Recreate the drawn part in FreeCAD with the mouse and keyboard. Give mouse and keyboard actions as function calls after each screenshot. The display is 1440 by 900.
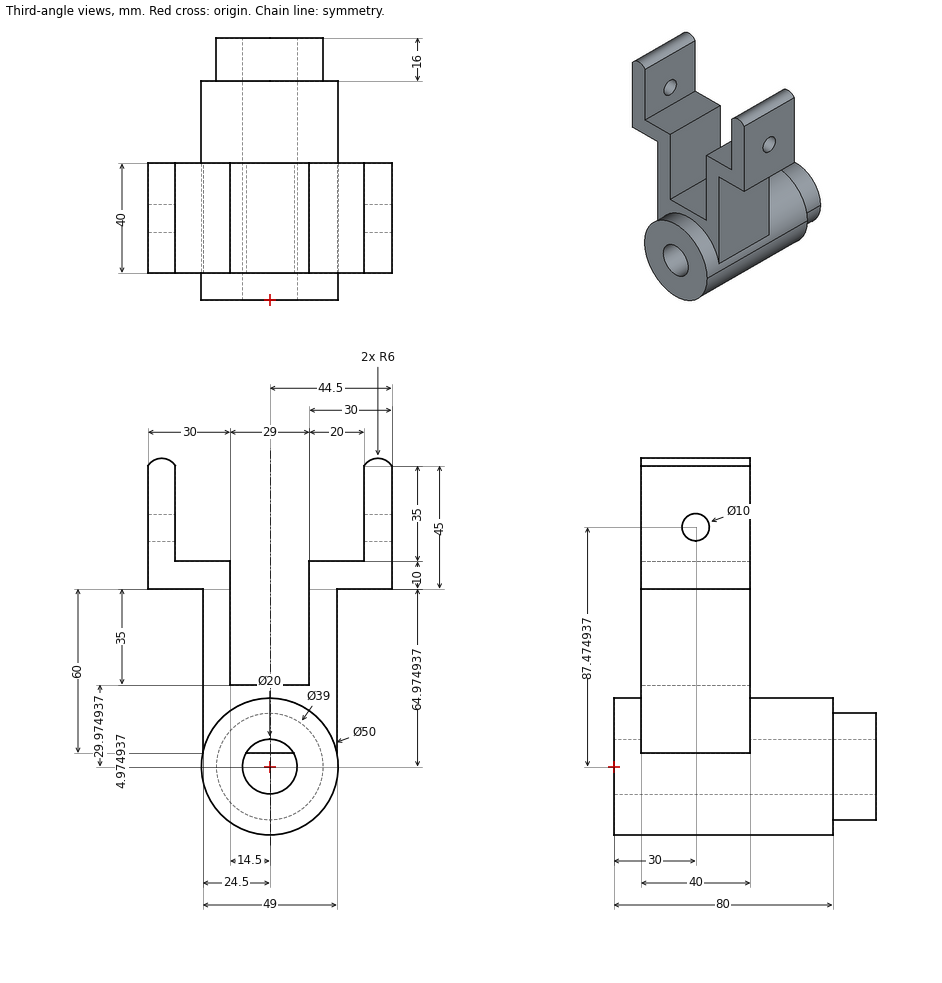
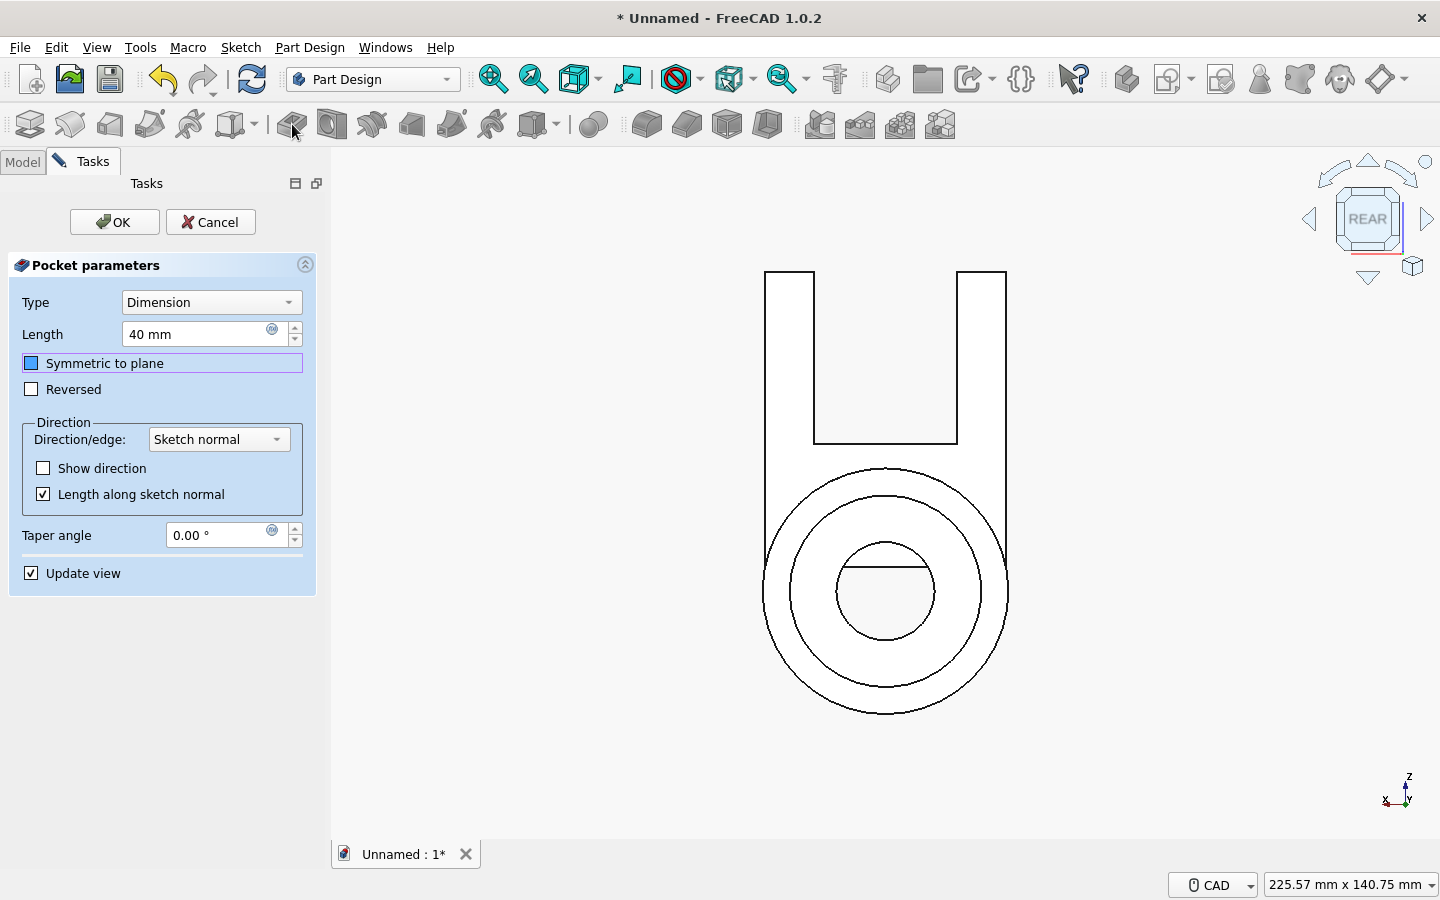
click(115, 222)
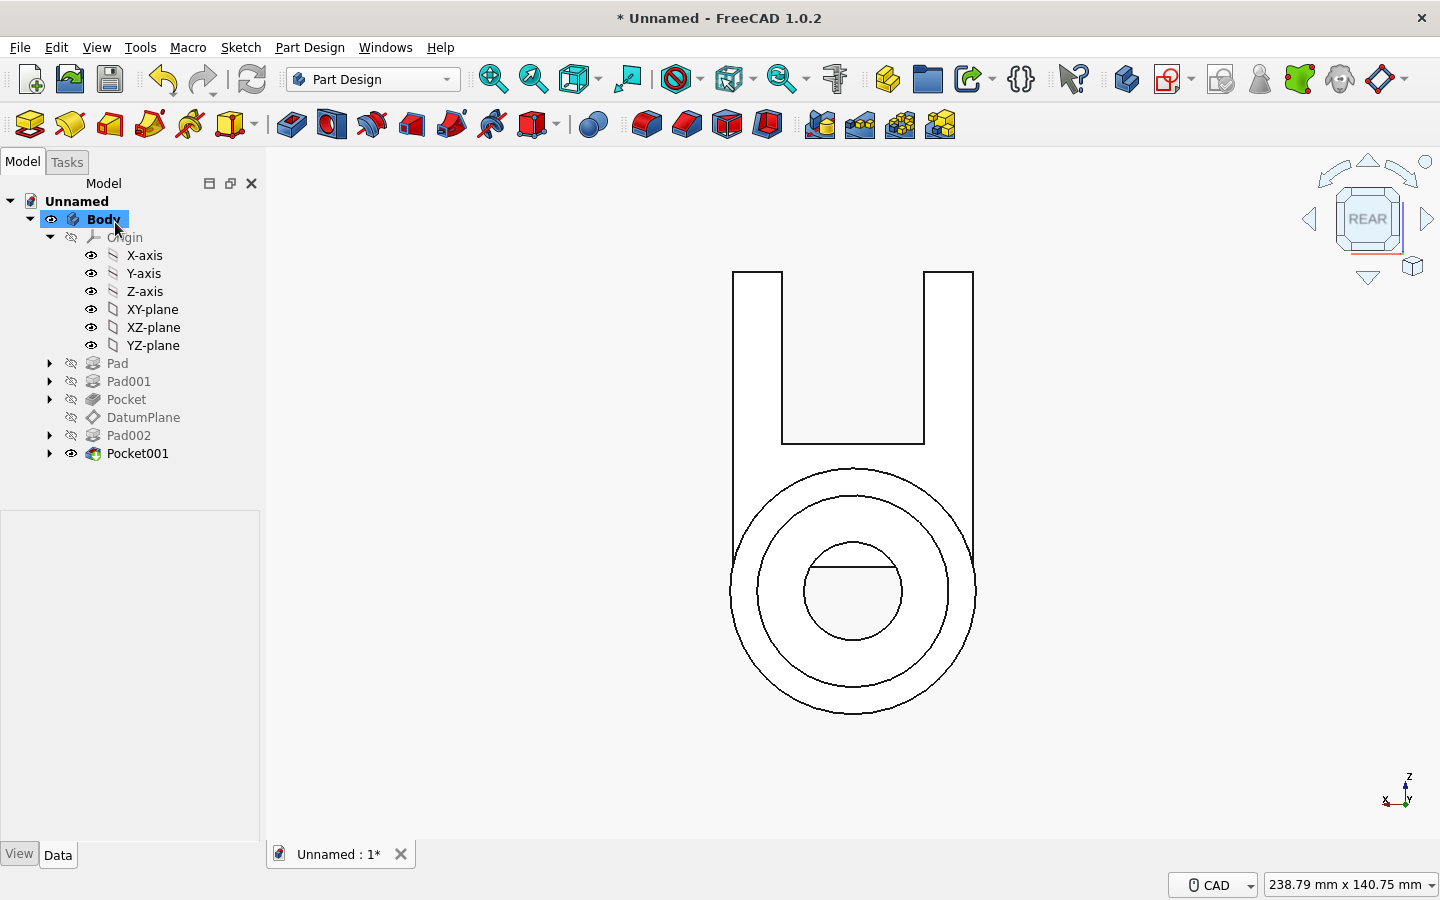
click(784, 460)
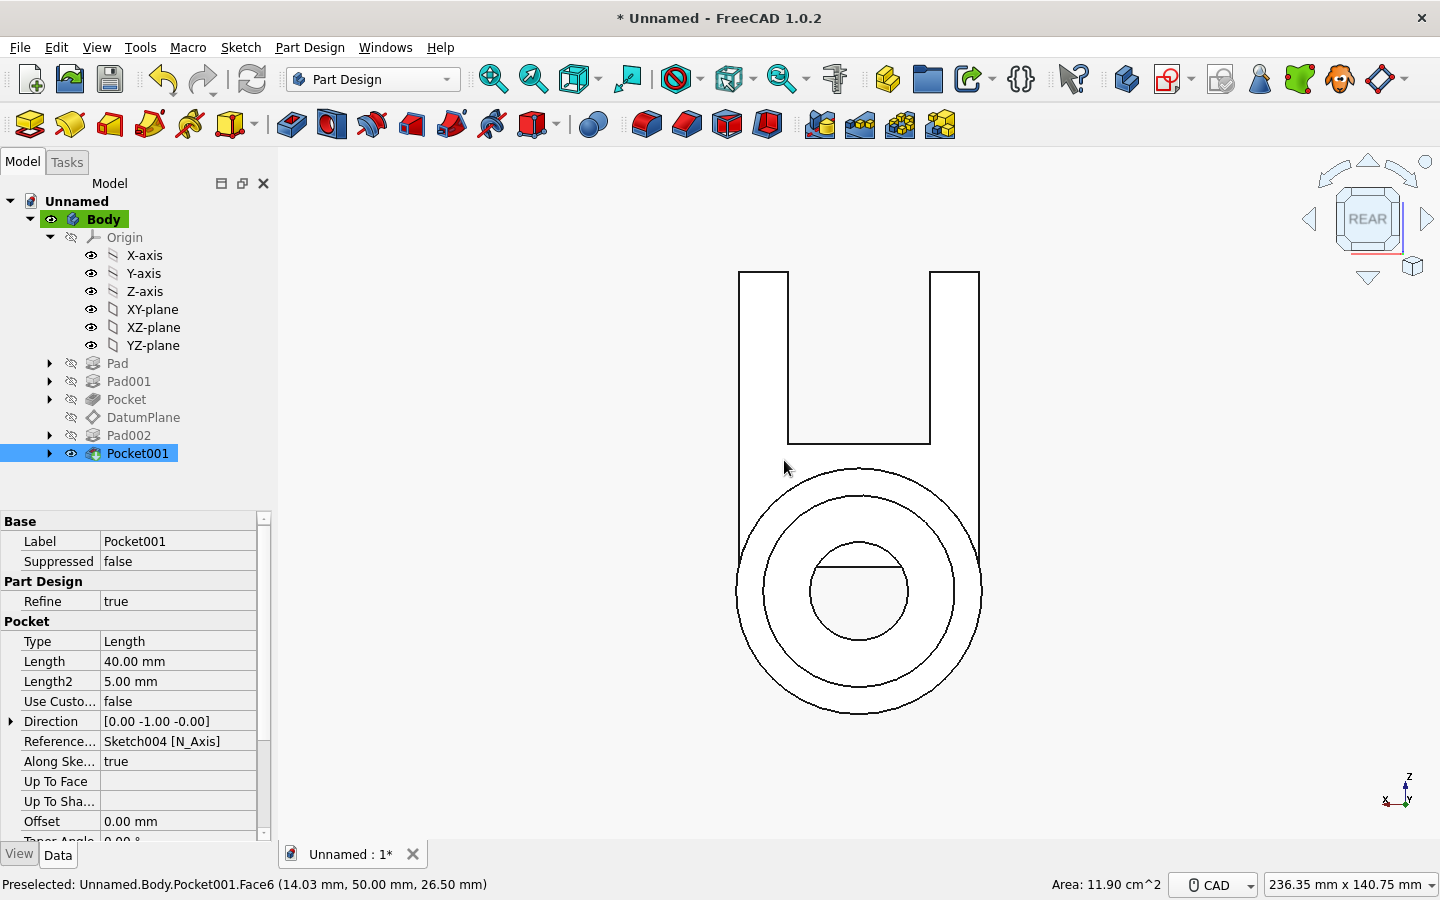
click(1168, 80)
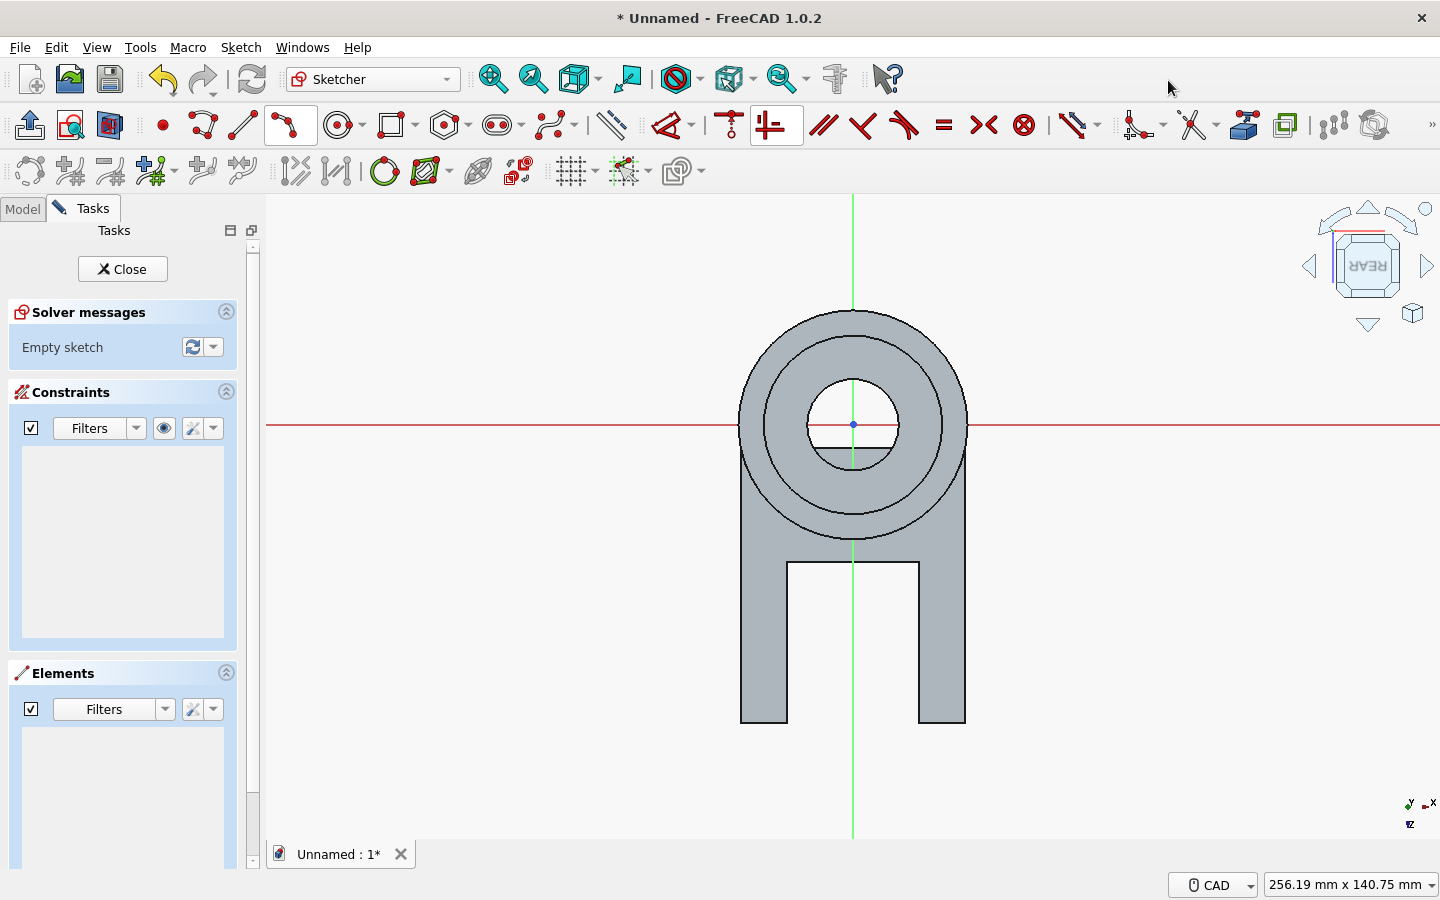
key(q)
key(s)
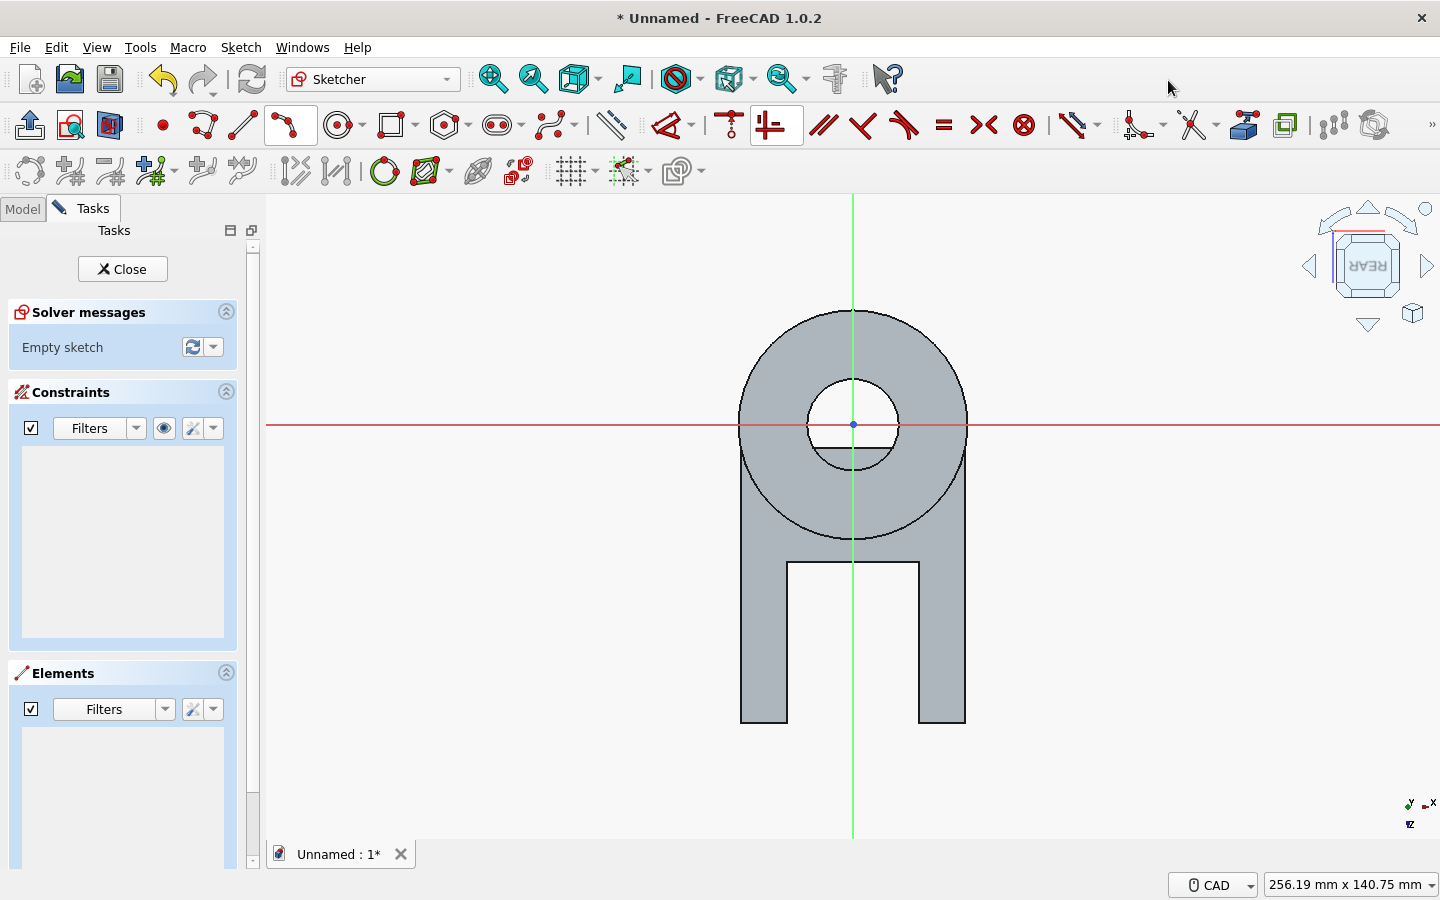
scroll(645, 222, down, 2)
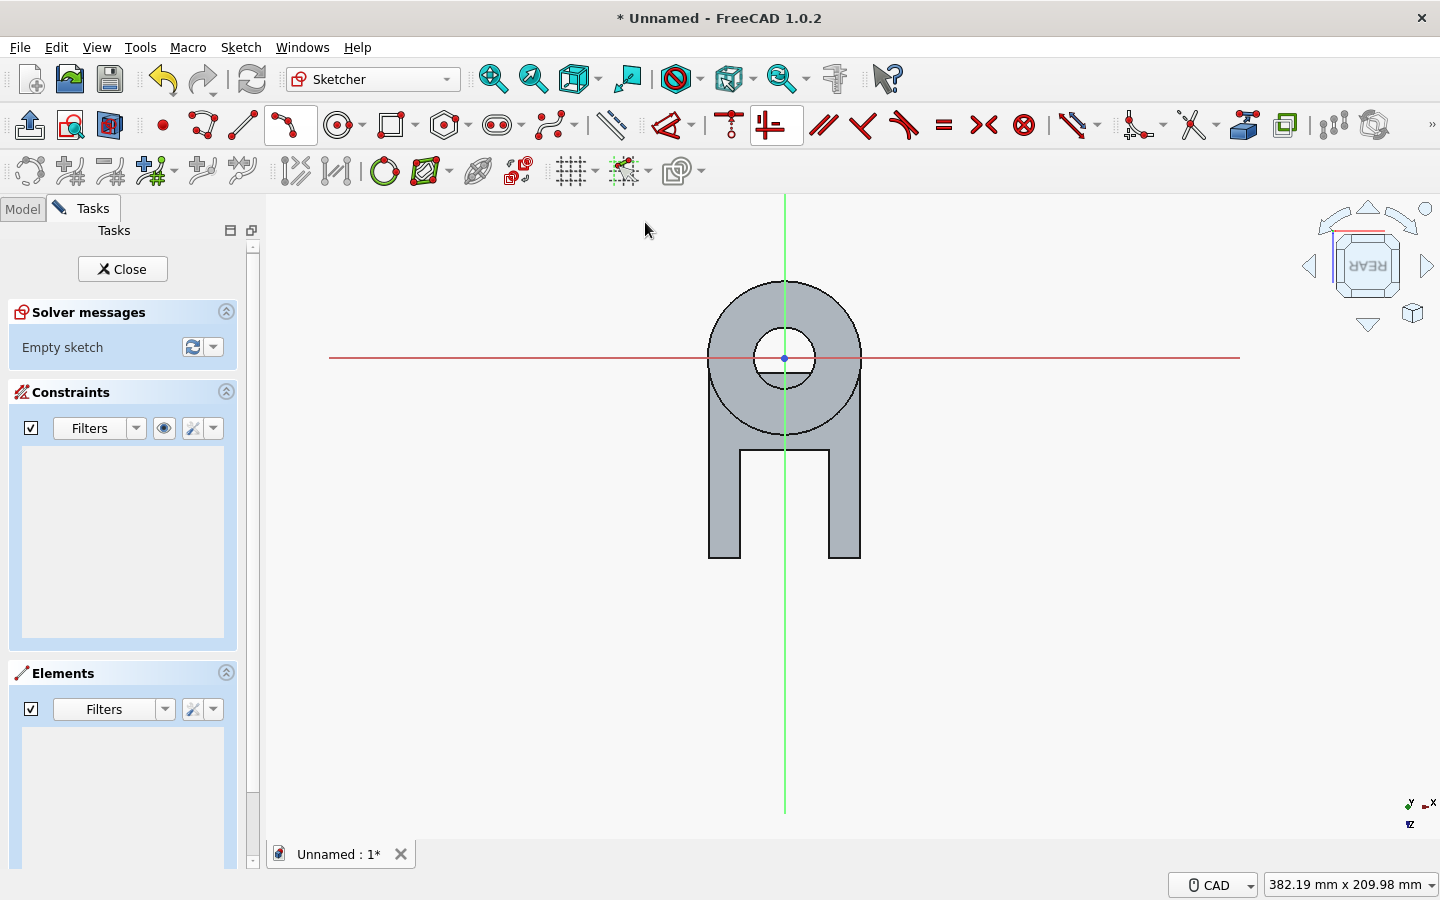
click(204, 126)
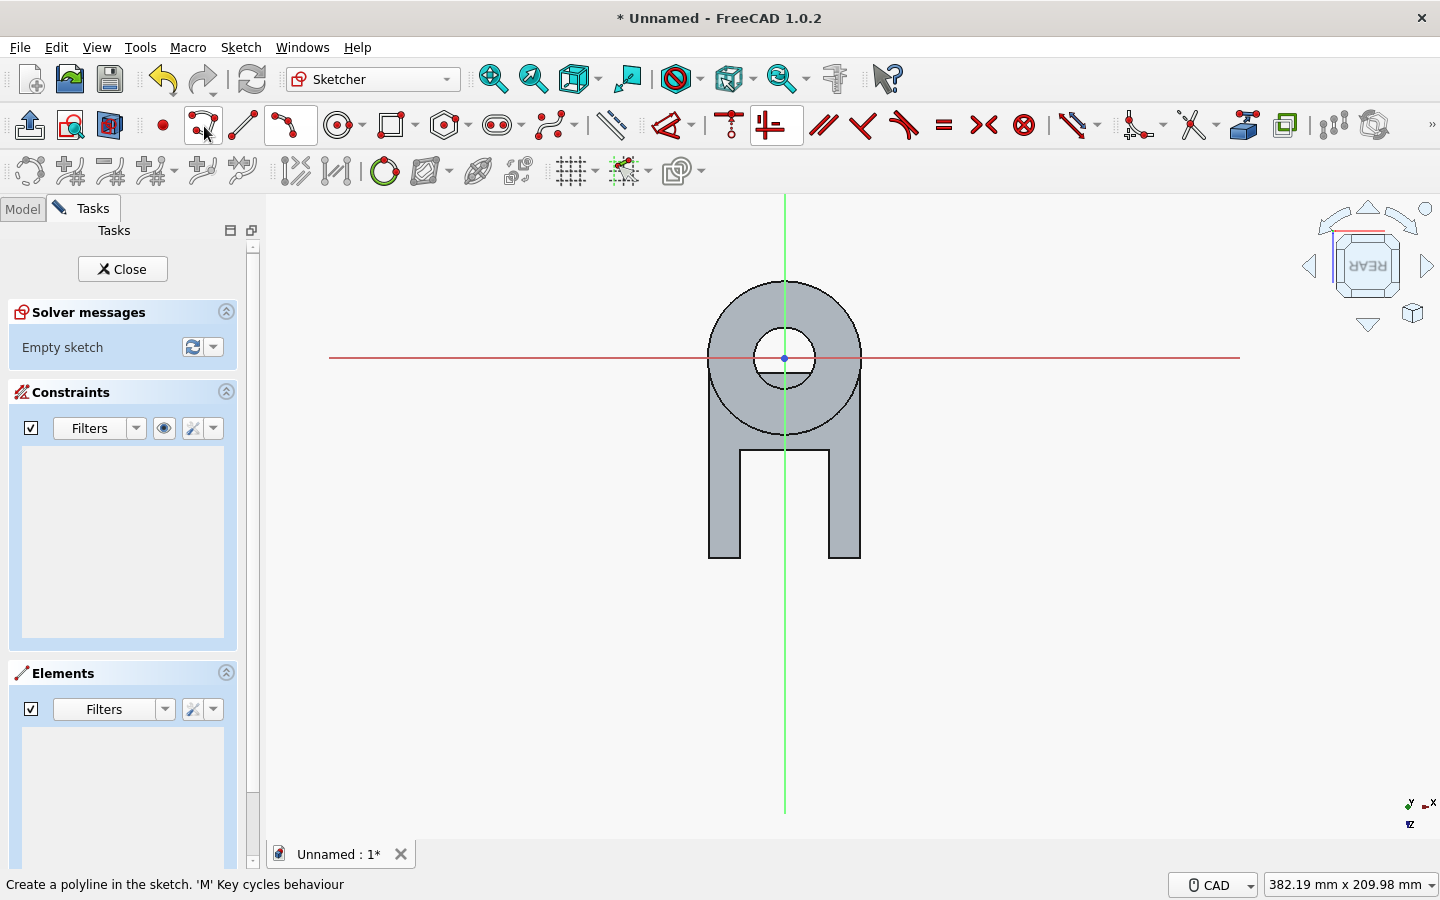
click(921, 696)
click(921, 558)
click(829, 558)
click(829, 588)
click(891, 588)
click(891, 696)
right_click(891, 696)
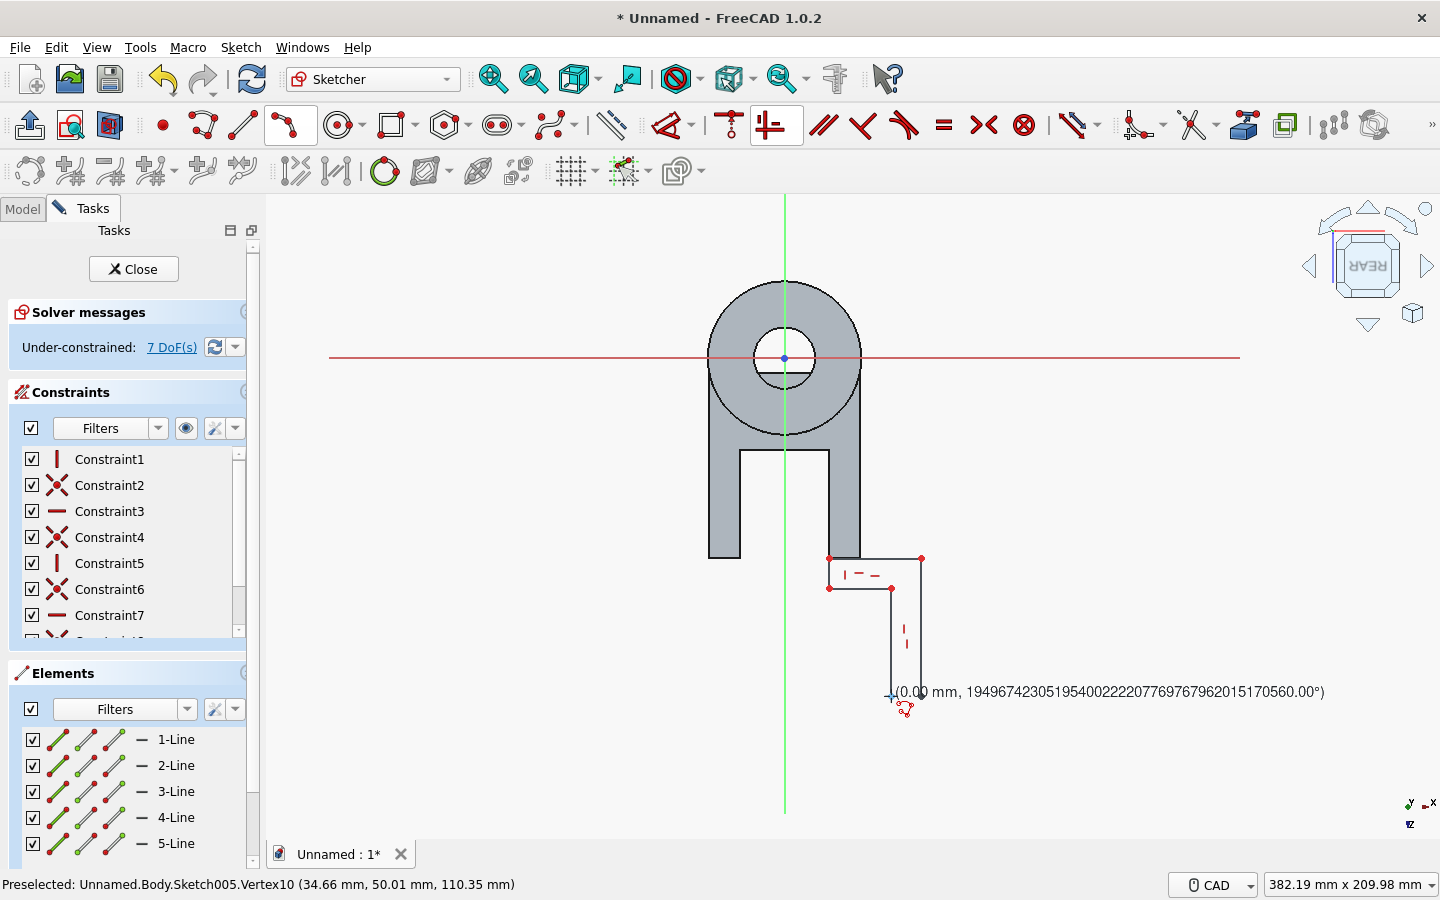
click(284, 126)